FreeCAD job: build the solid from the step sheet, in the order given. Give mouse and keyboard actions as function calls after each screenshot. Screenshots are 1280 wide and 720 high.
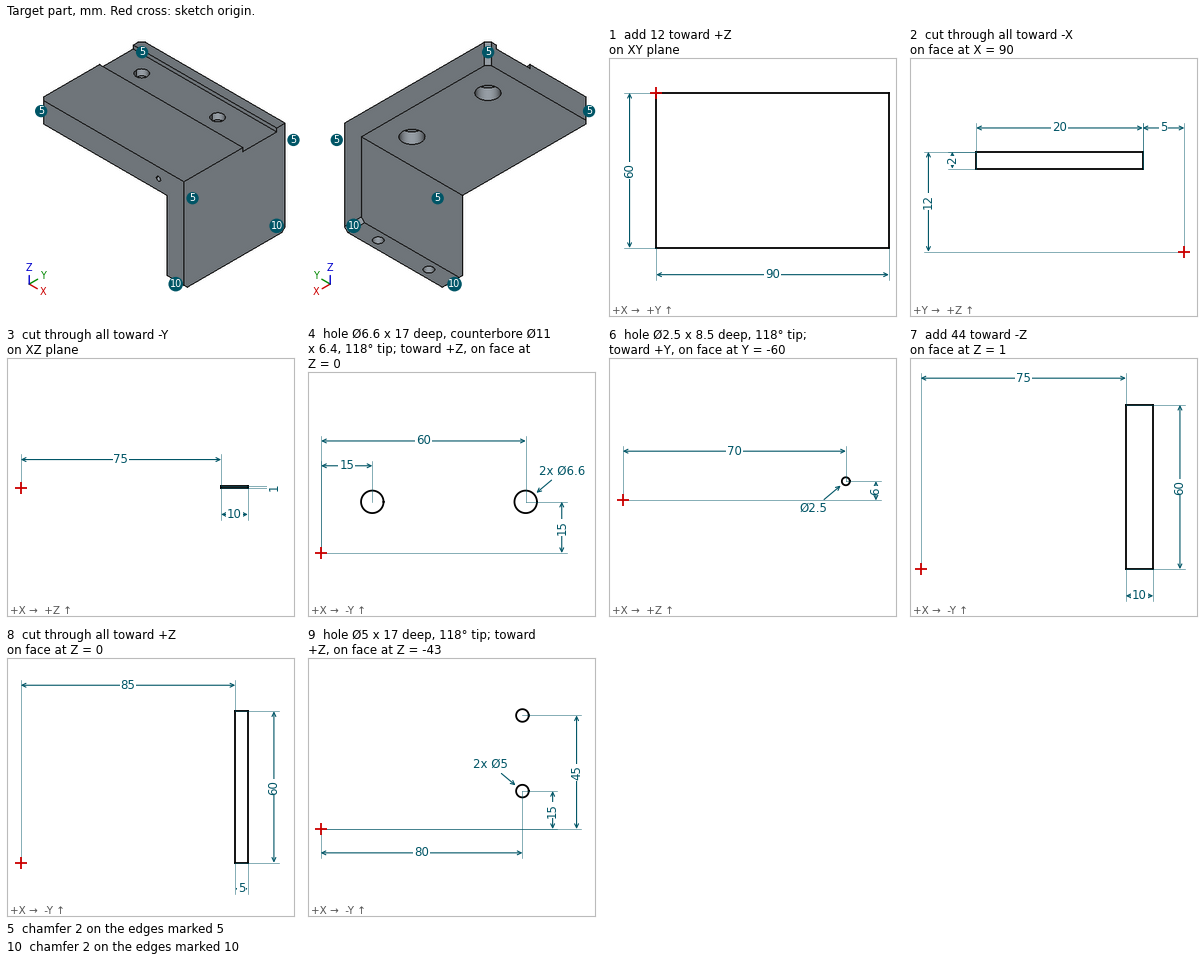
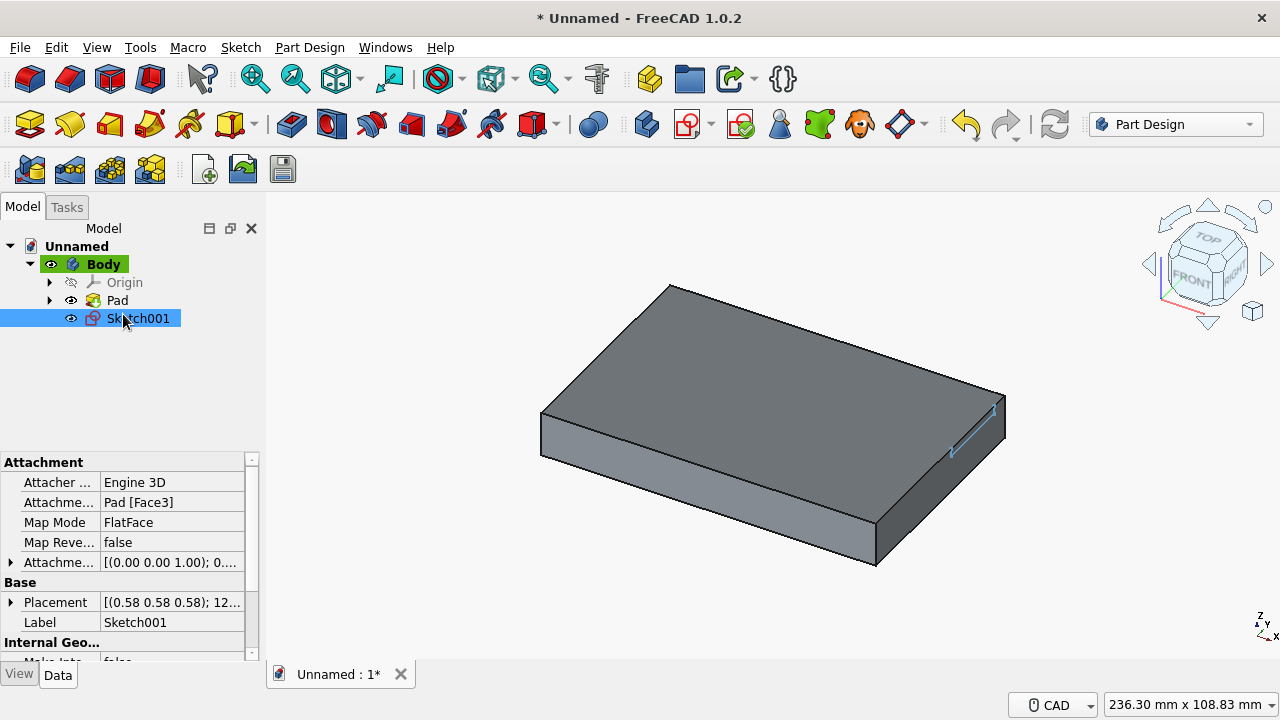
click(292, 124)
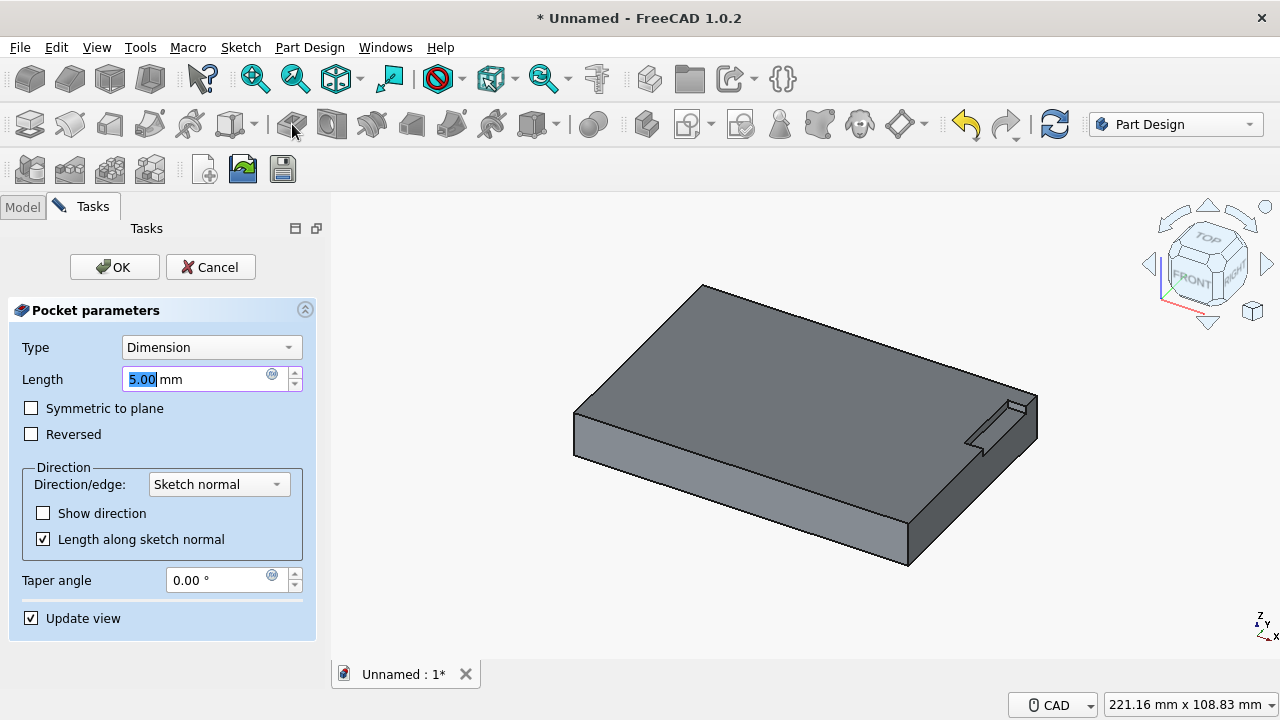
click(212, 348)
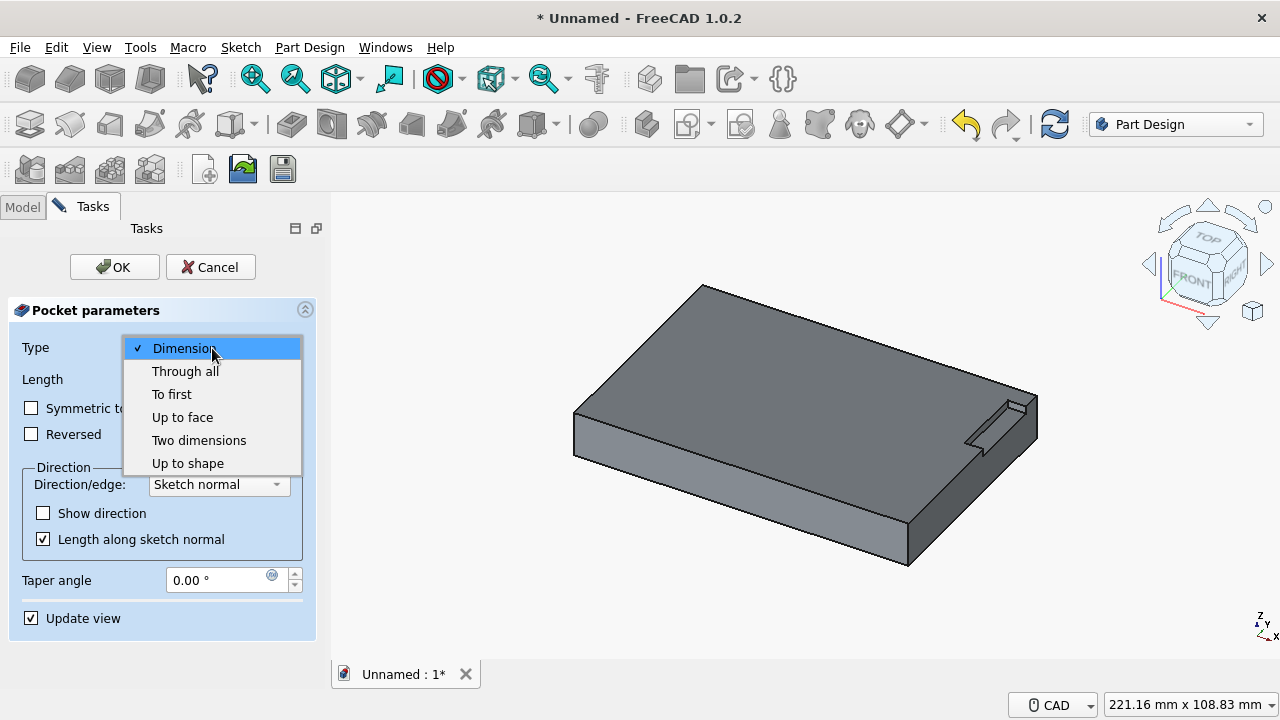
click(212, 372)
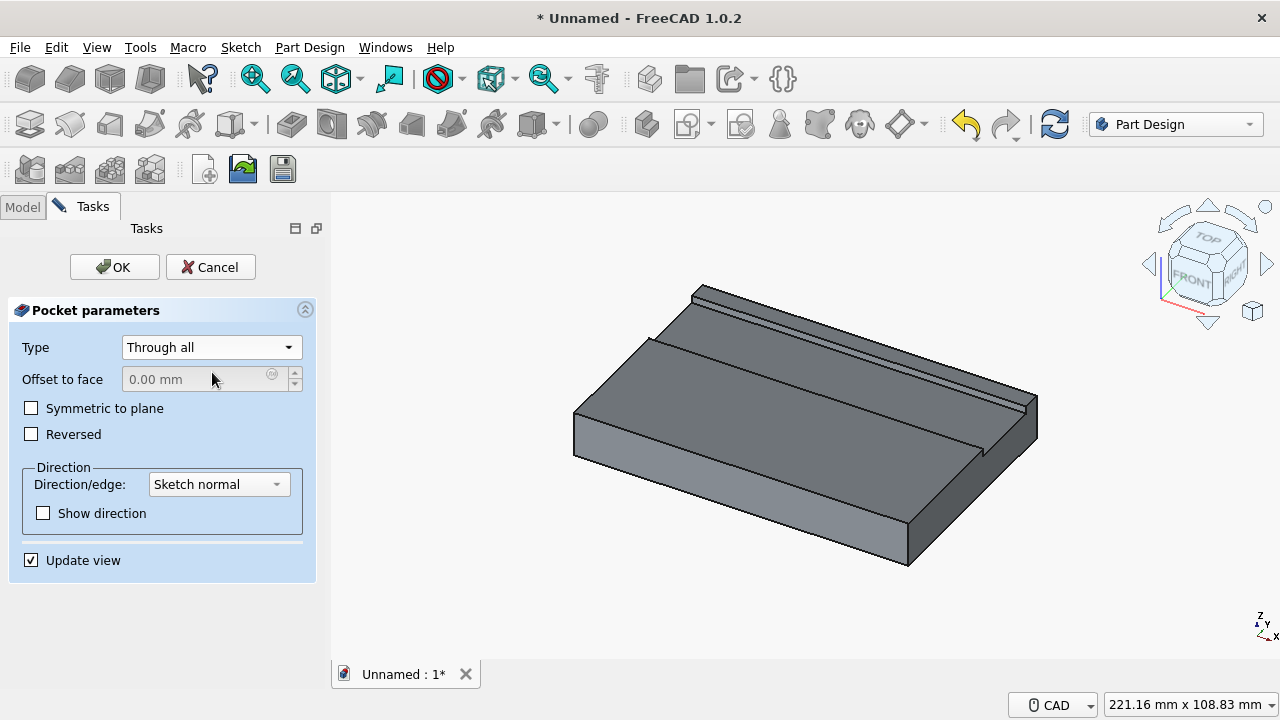
click(115, 267)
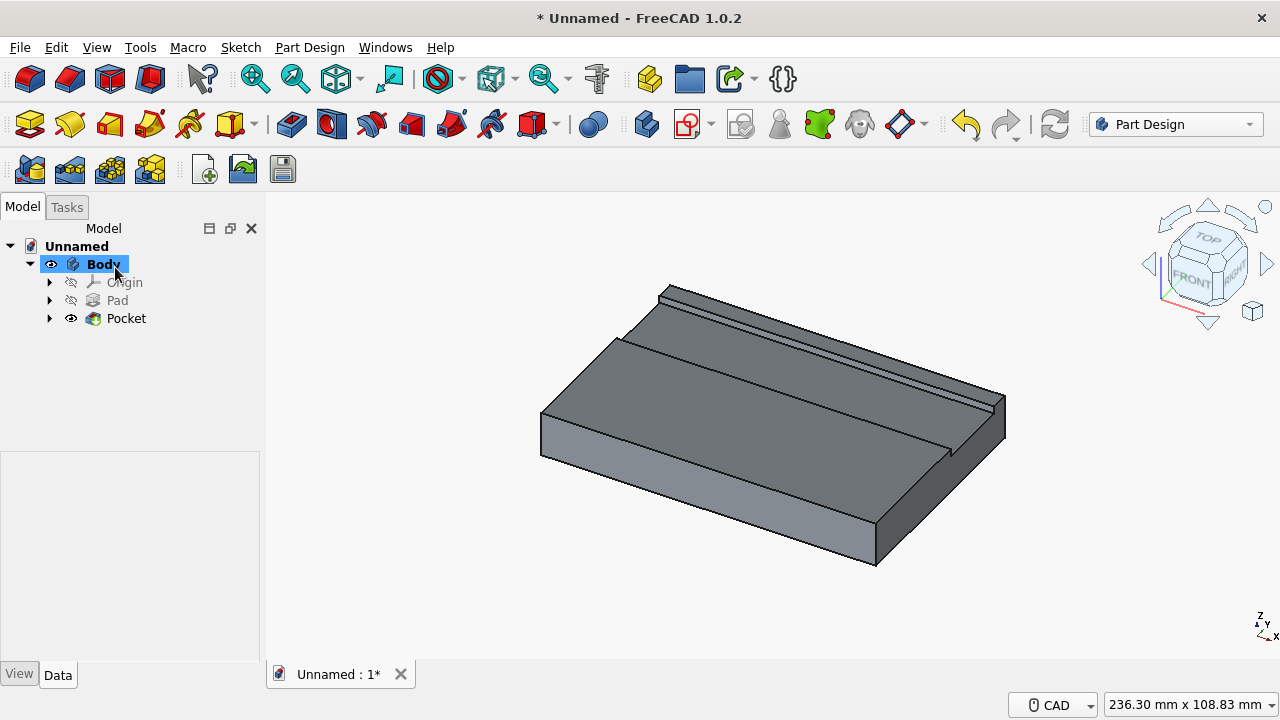
click(688, 124)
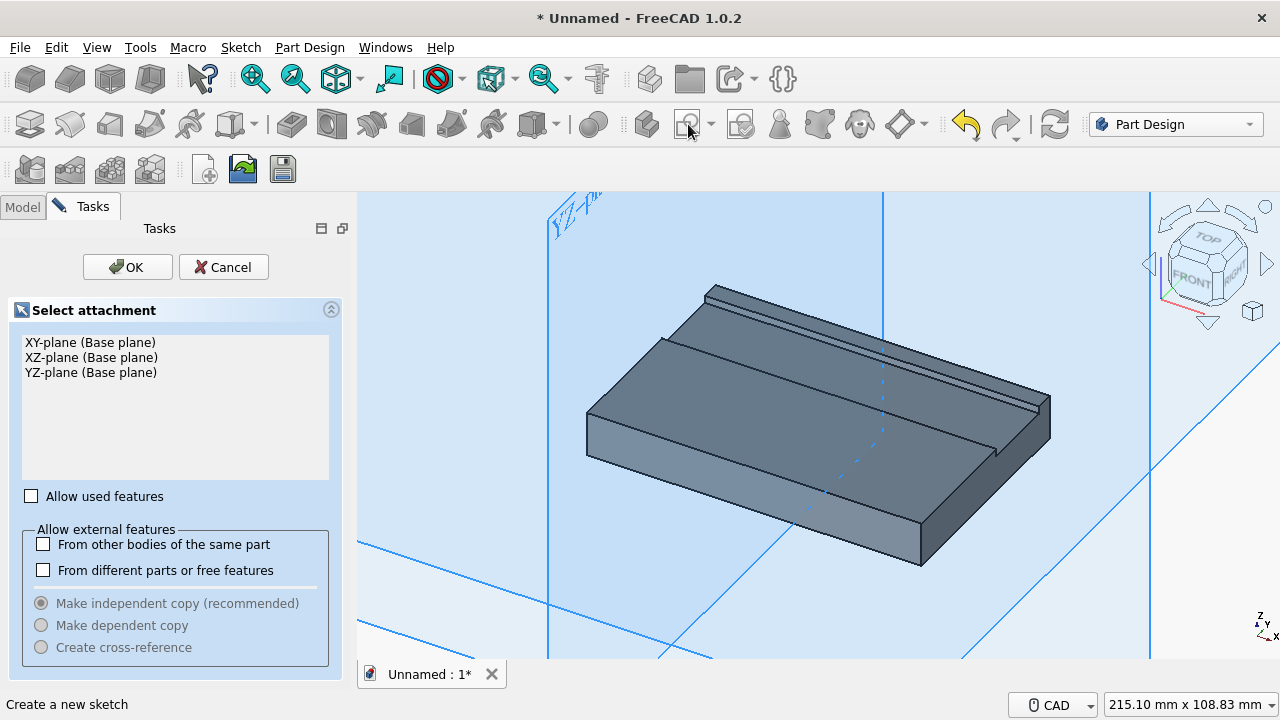
click(82, 358)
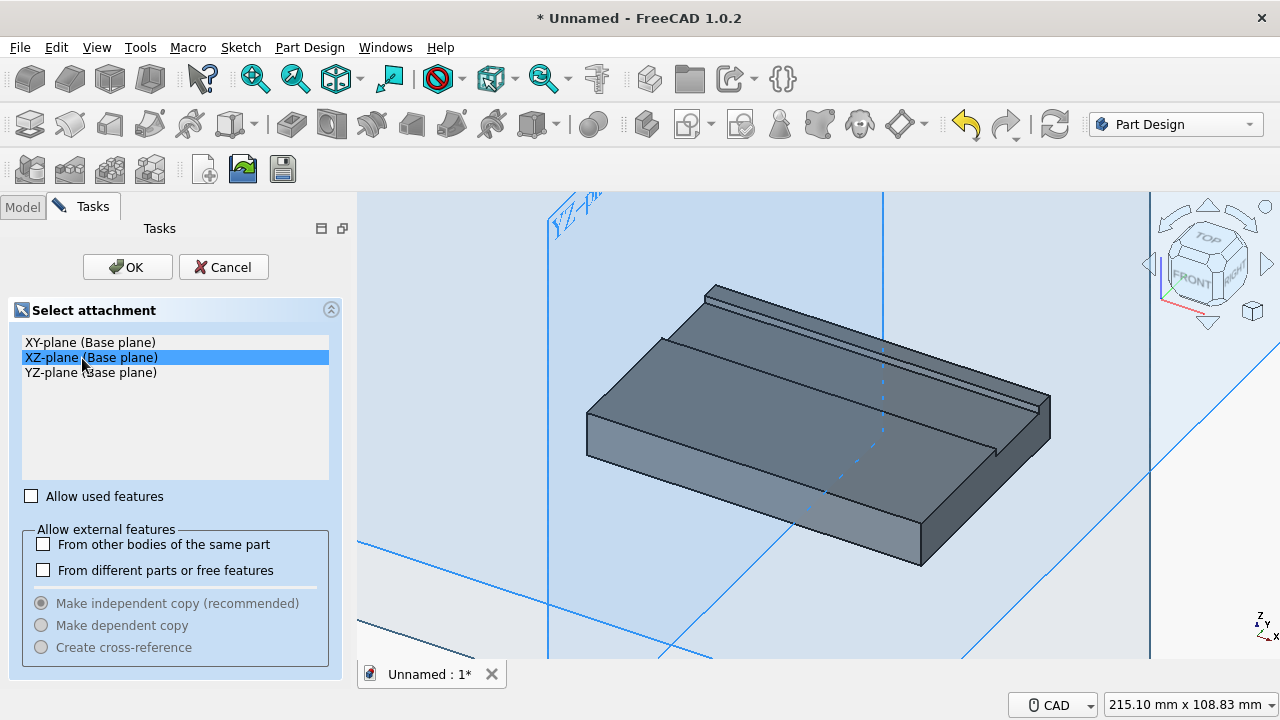
click(128, 267)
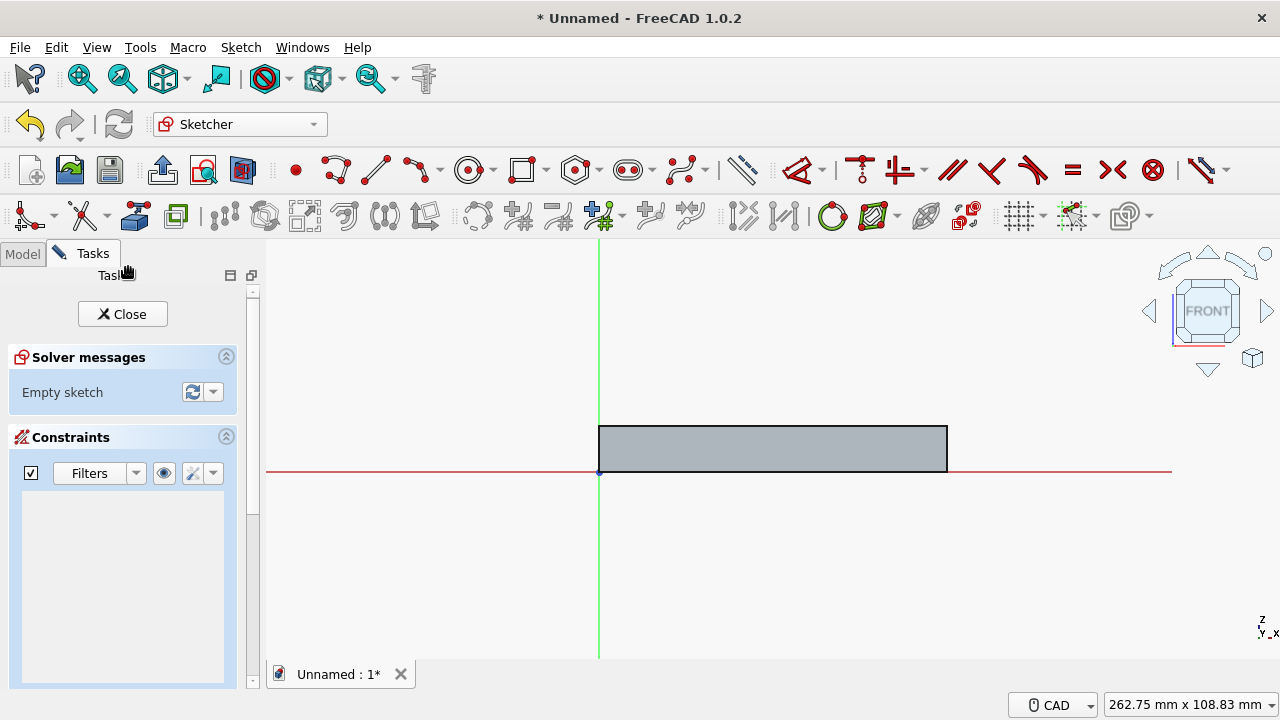
click(244, 170)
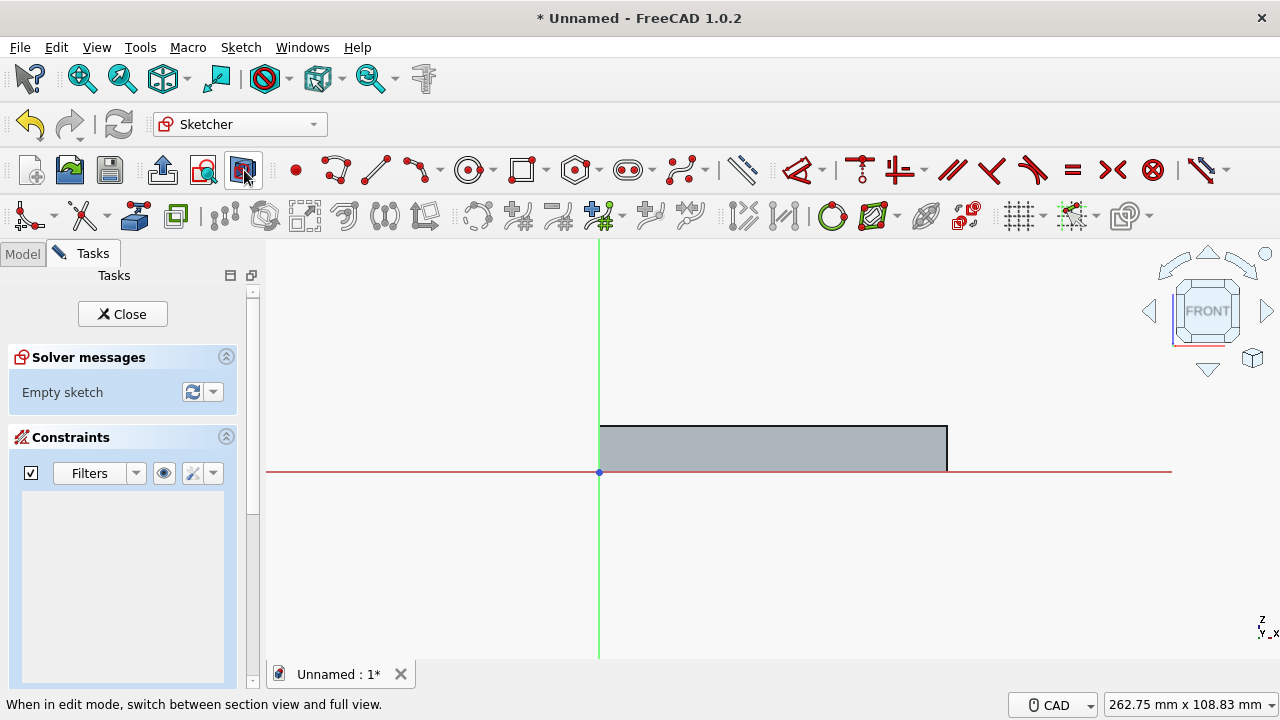
scroll(921, 472, up, 14)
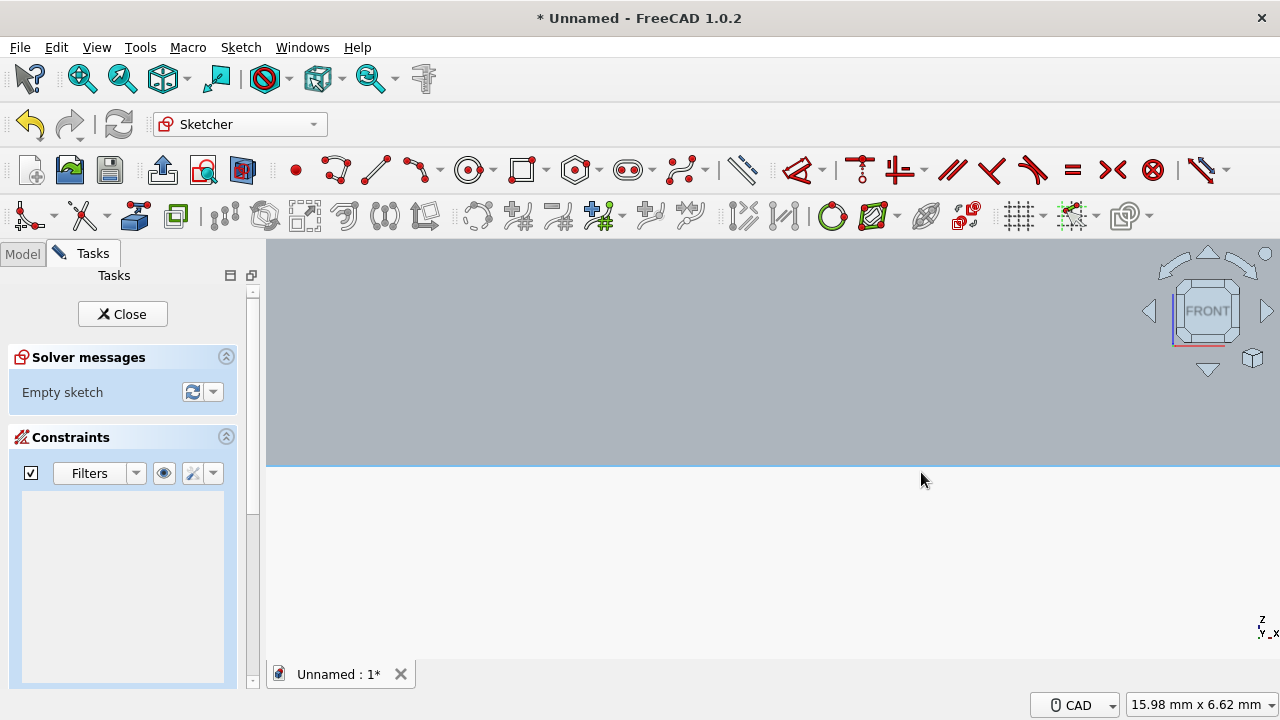
click(522, 170)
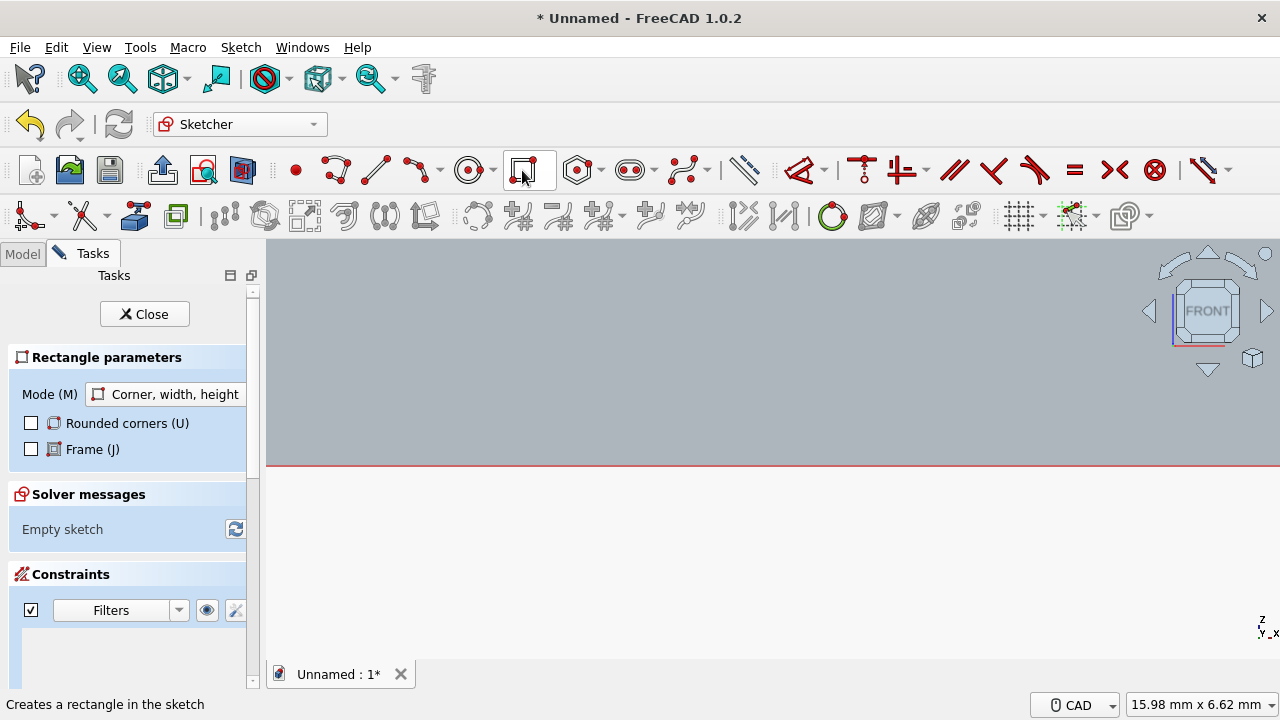
click(381, 403)
click(1016, 466)
key(Escape)